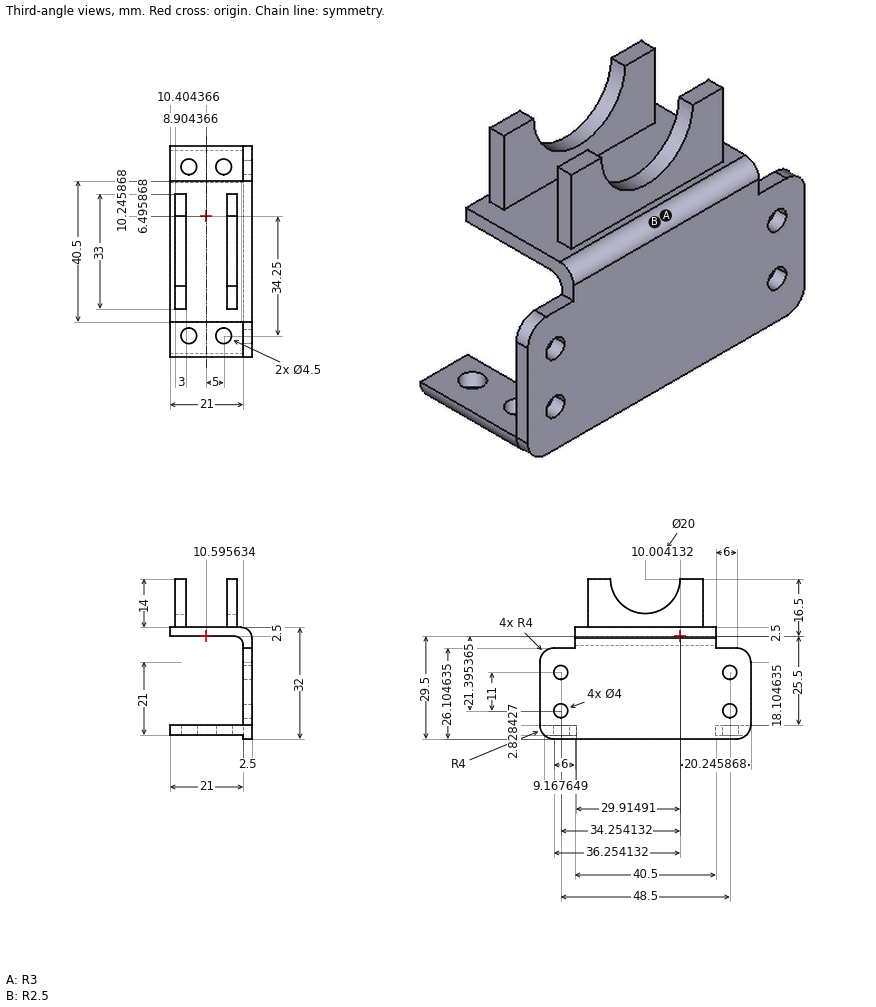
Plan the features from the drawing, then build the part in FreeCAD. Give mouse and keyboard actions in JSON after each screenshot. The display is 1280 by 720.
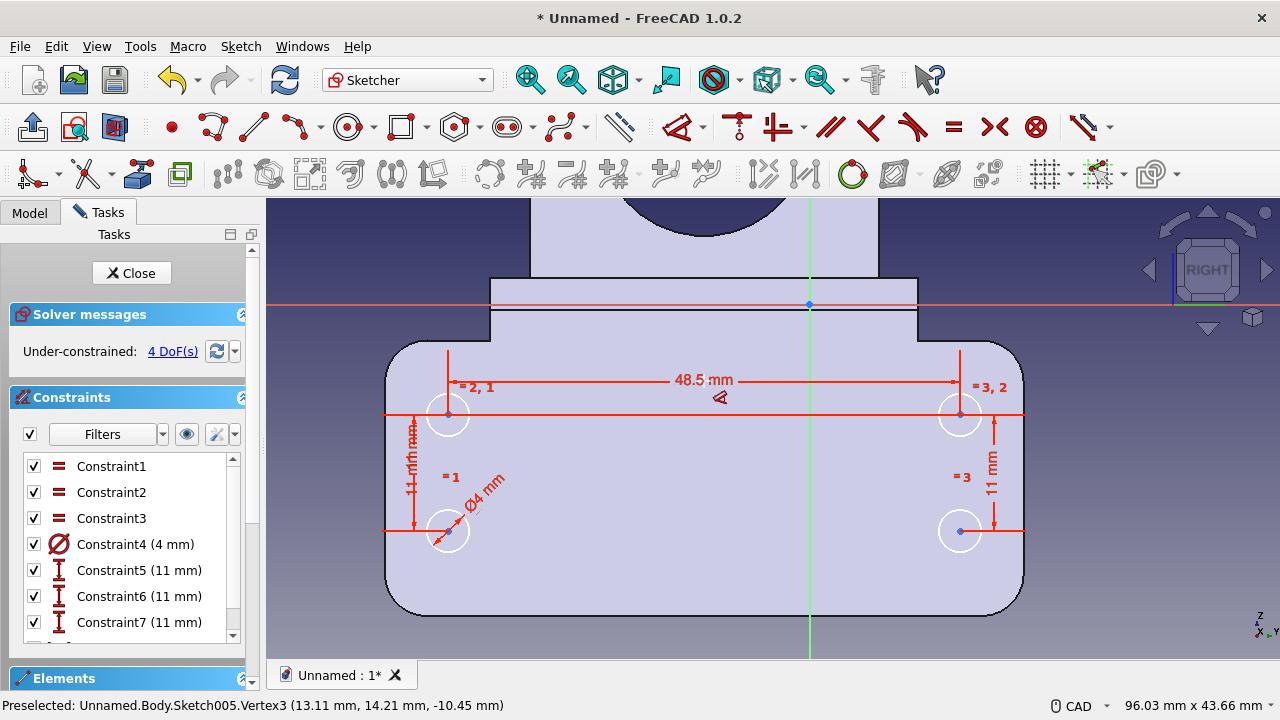
{"action": "left_click", "coordinate": [448, 531]}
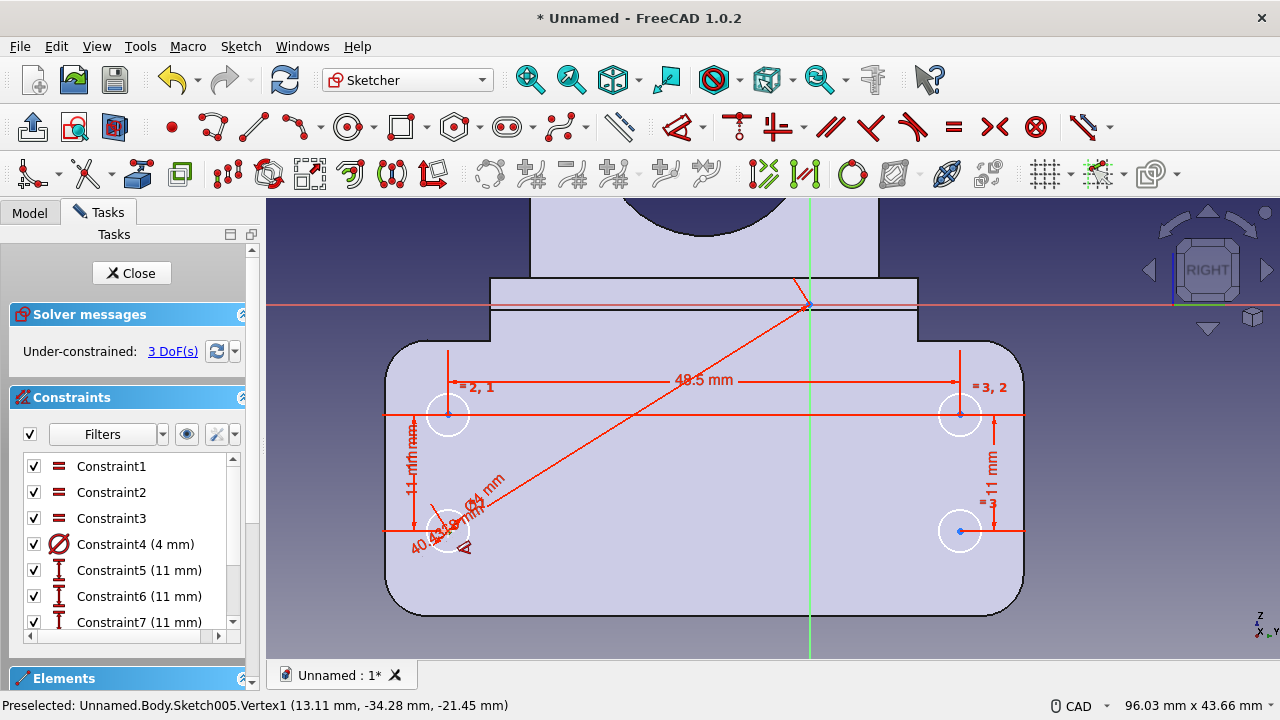
{"action": "left_click", "coordinate": [960, 415]}
{"action": "left_click", "coordinate": [704, 565]}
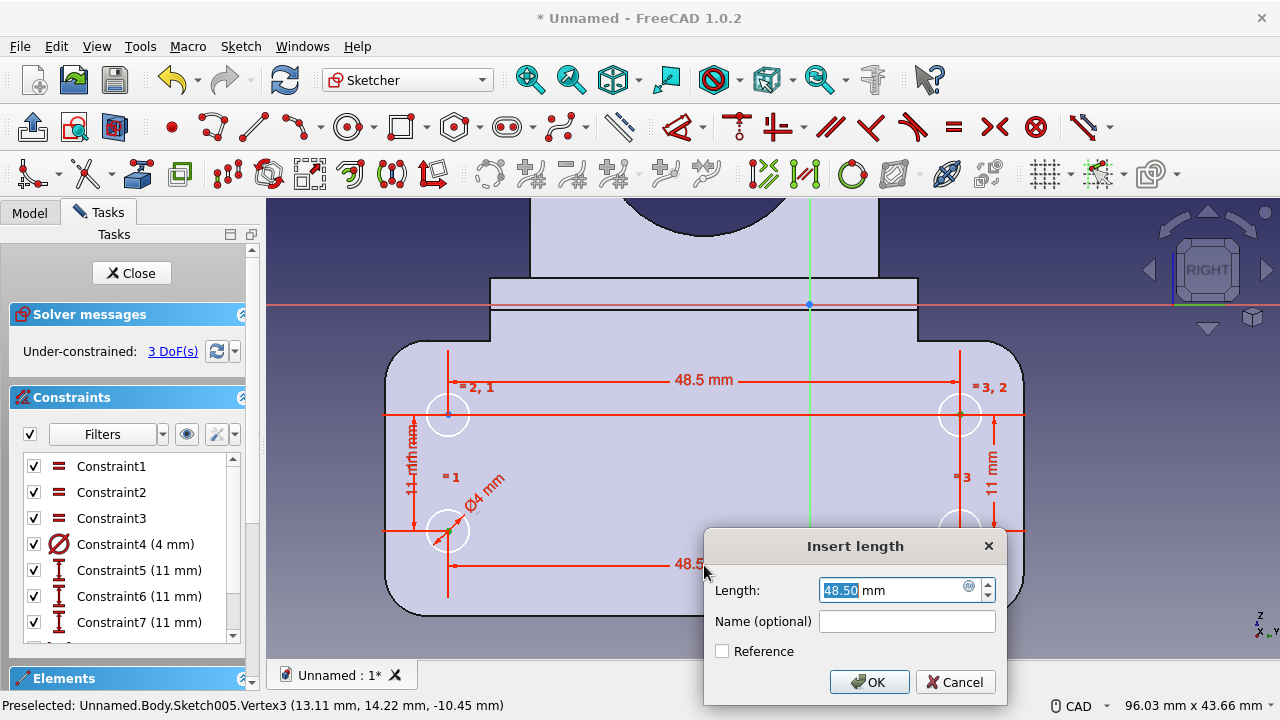
{"action": "type", "text": "48.5"}
{"action": "key", "text": "Return"}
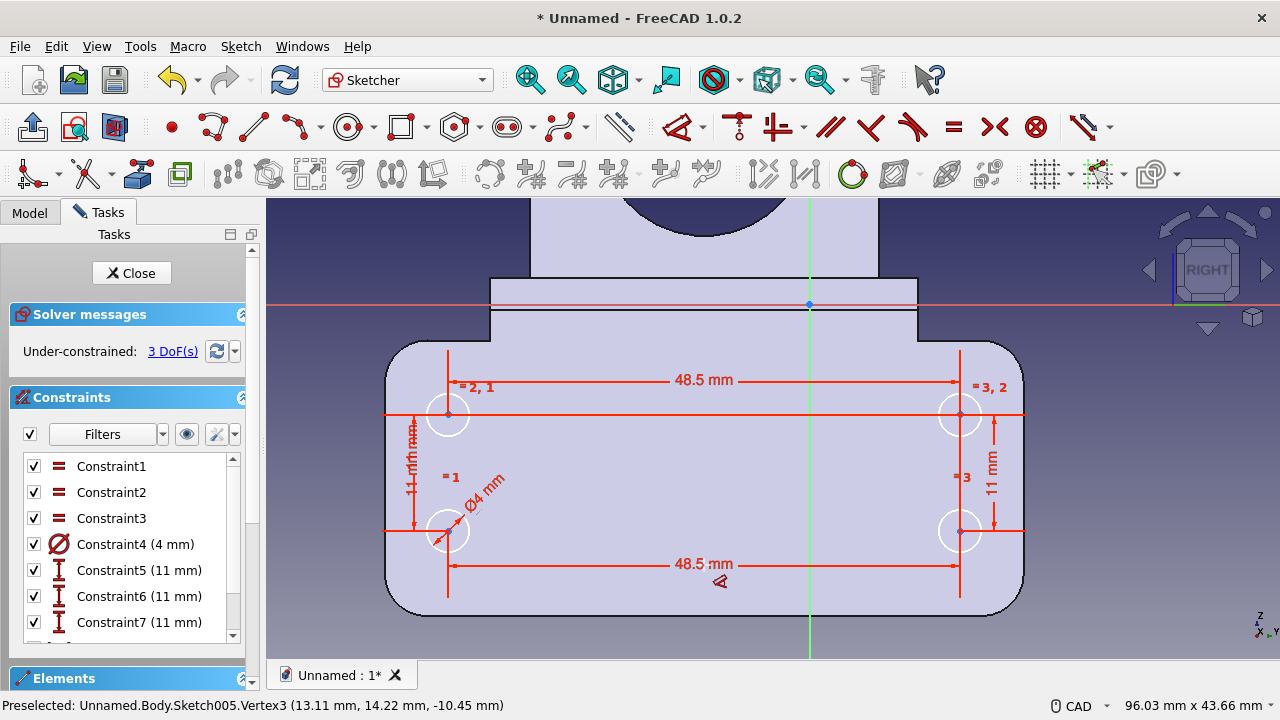
{"action": "left_click", "coordinate": [448, 531]}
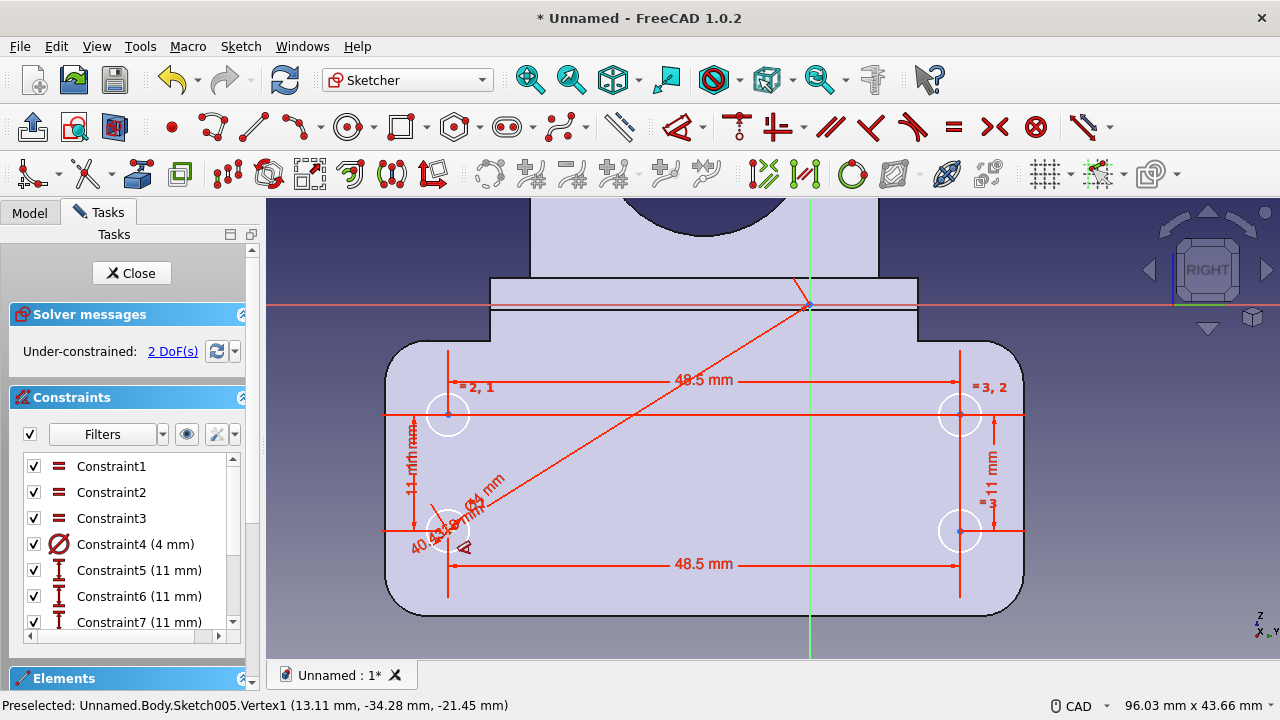
{"action": "left_click", "coordinate": [960, 531]}
{"action": "left_click", "coordinate": [586, 565]}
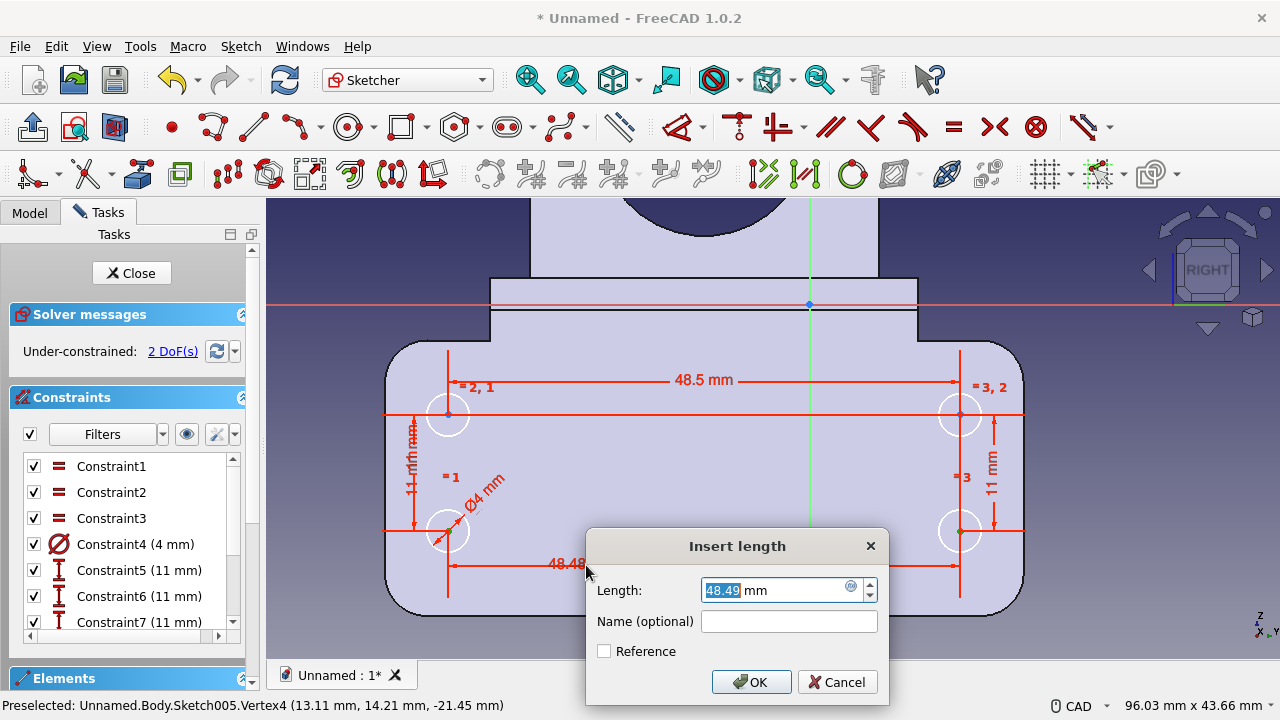
{"action": "type", "text": "48.5"}
{"action": "key", "text": "Return"}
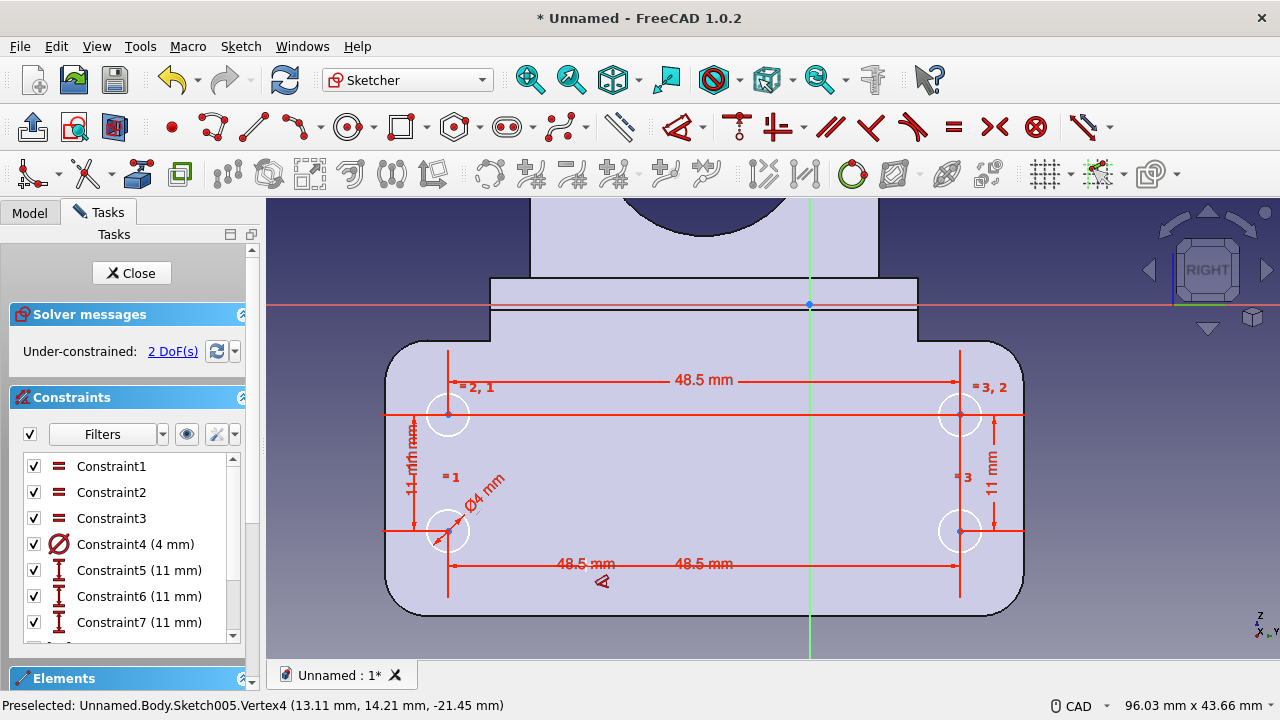
{"action": "left_click", "coordinate": [448, 531]}
{"action": "left_click", "coordinate": [629, 271]}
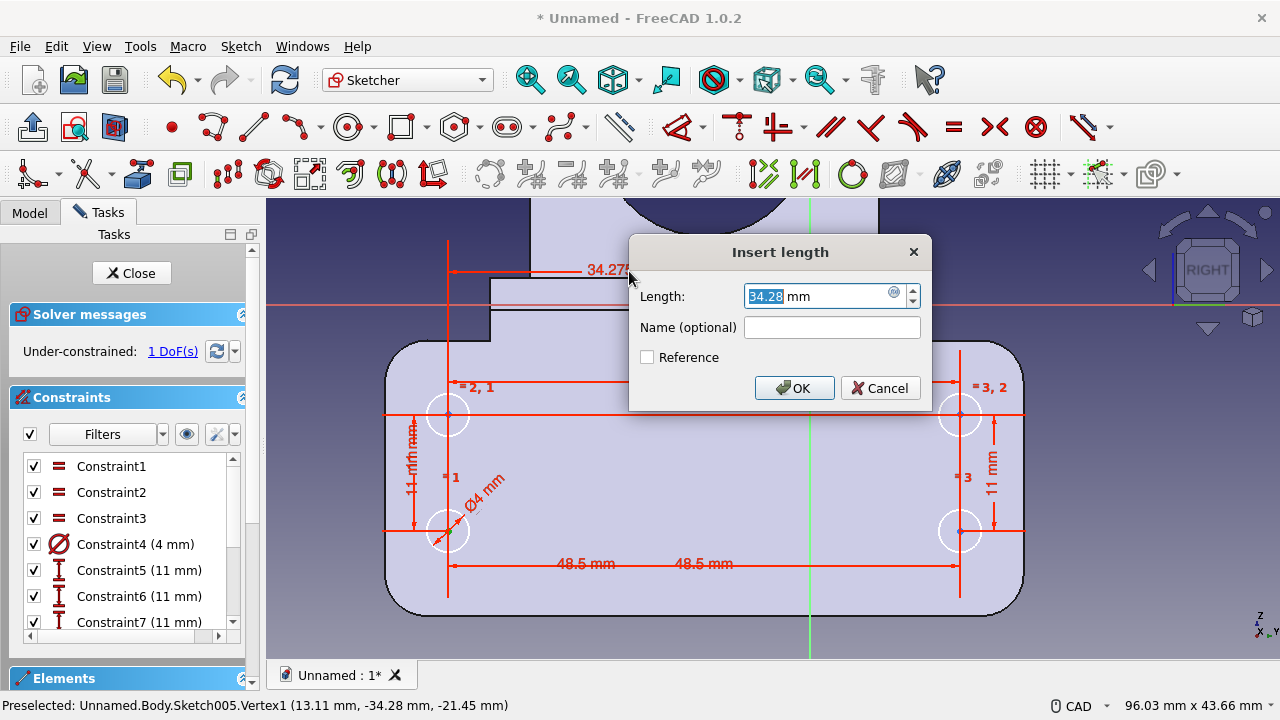
{"action": "type", "text": "34.254132"}
{"action": "key", "text": "Return"}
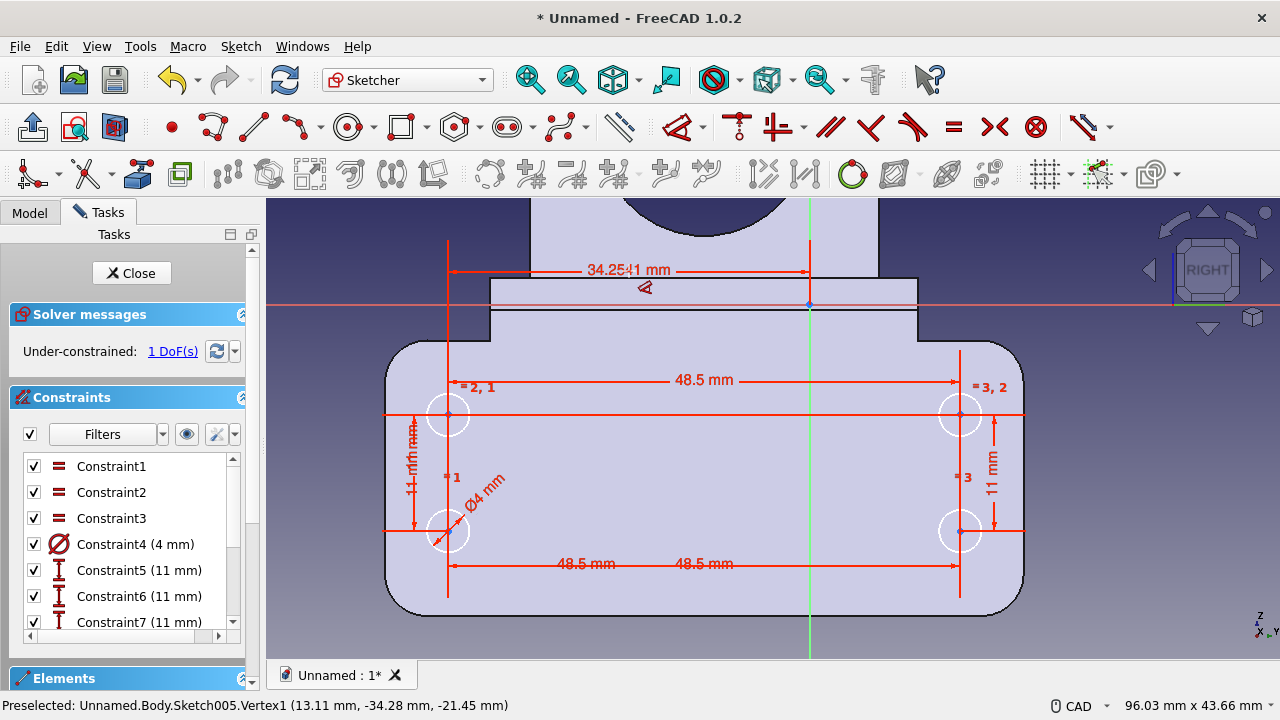
{"action": "left_click", "coordinate": [448, 531]}
{"action": "left_click", "coordinate": [414, 418]}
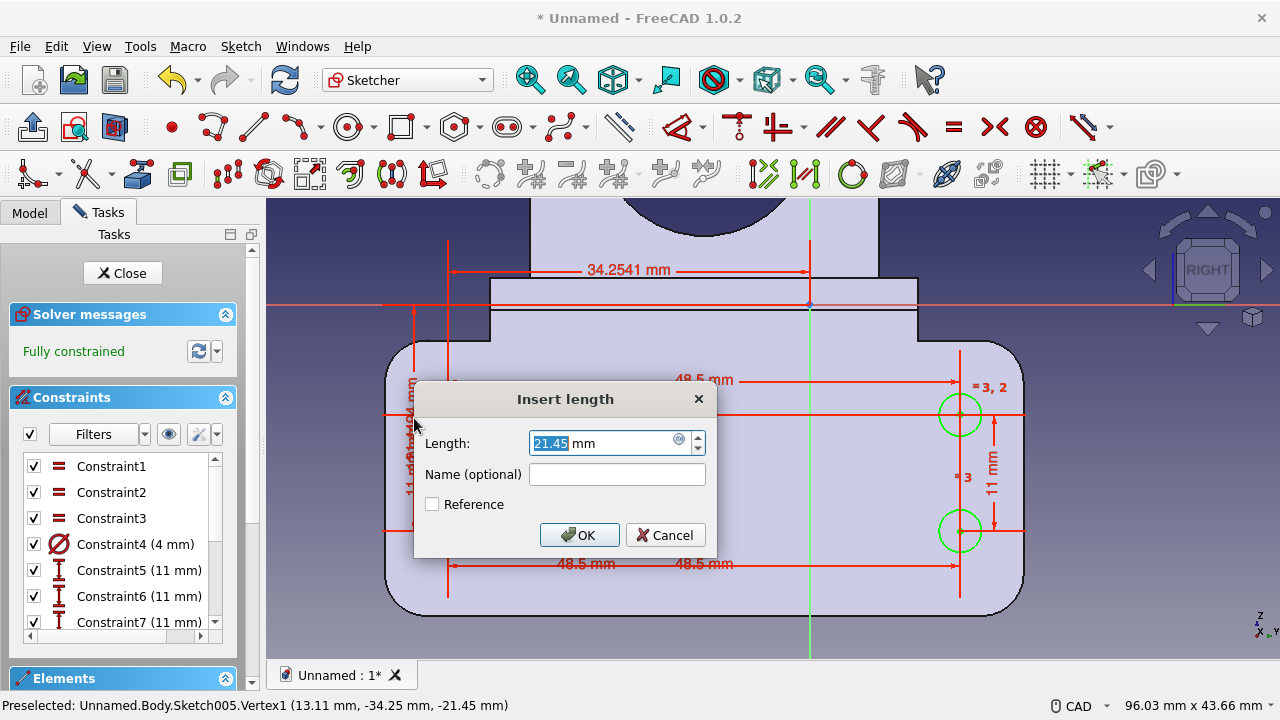
{"action": "type", "text": "21.395365"}
{"action": "key", "text": "Return"}
{"action": "key", "text": "Escape"}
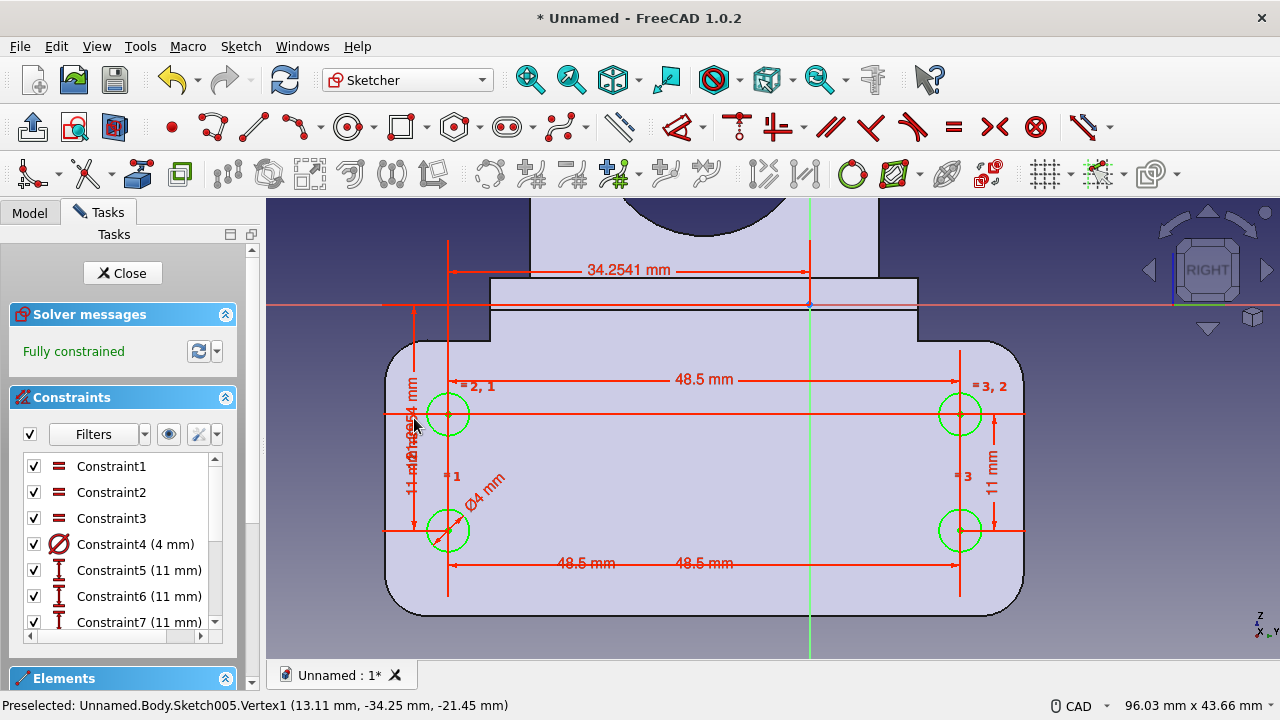
{"action": "left_click", "coordinate": [123, 273]}